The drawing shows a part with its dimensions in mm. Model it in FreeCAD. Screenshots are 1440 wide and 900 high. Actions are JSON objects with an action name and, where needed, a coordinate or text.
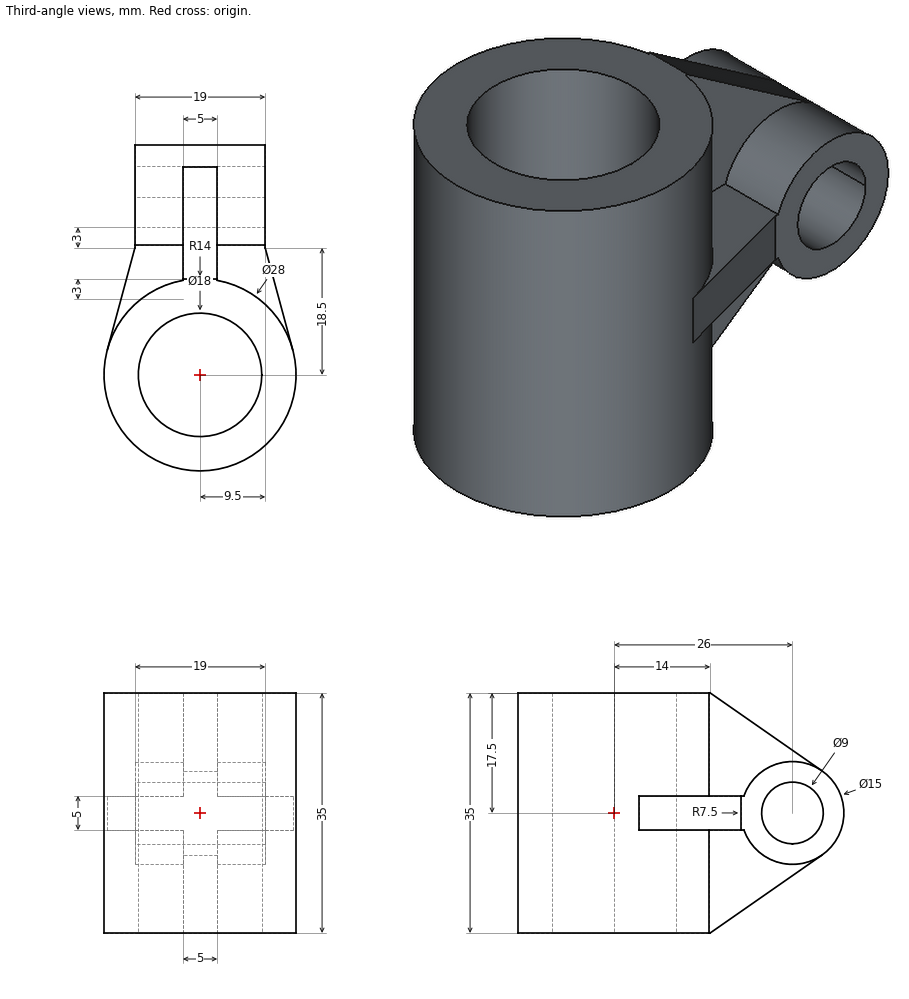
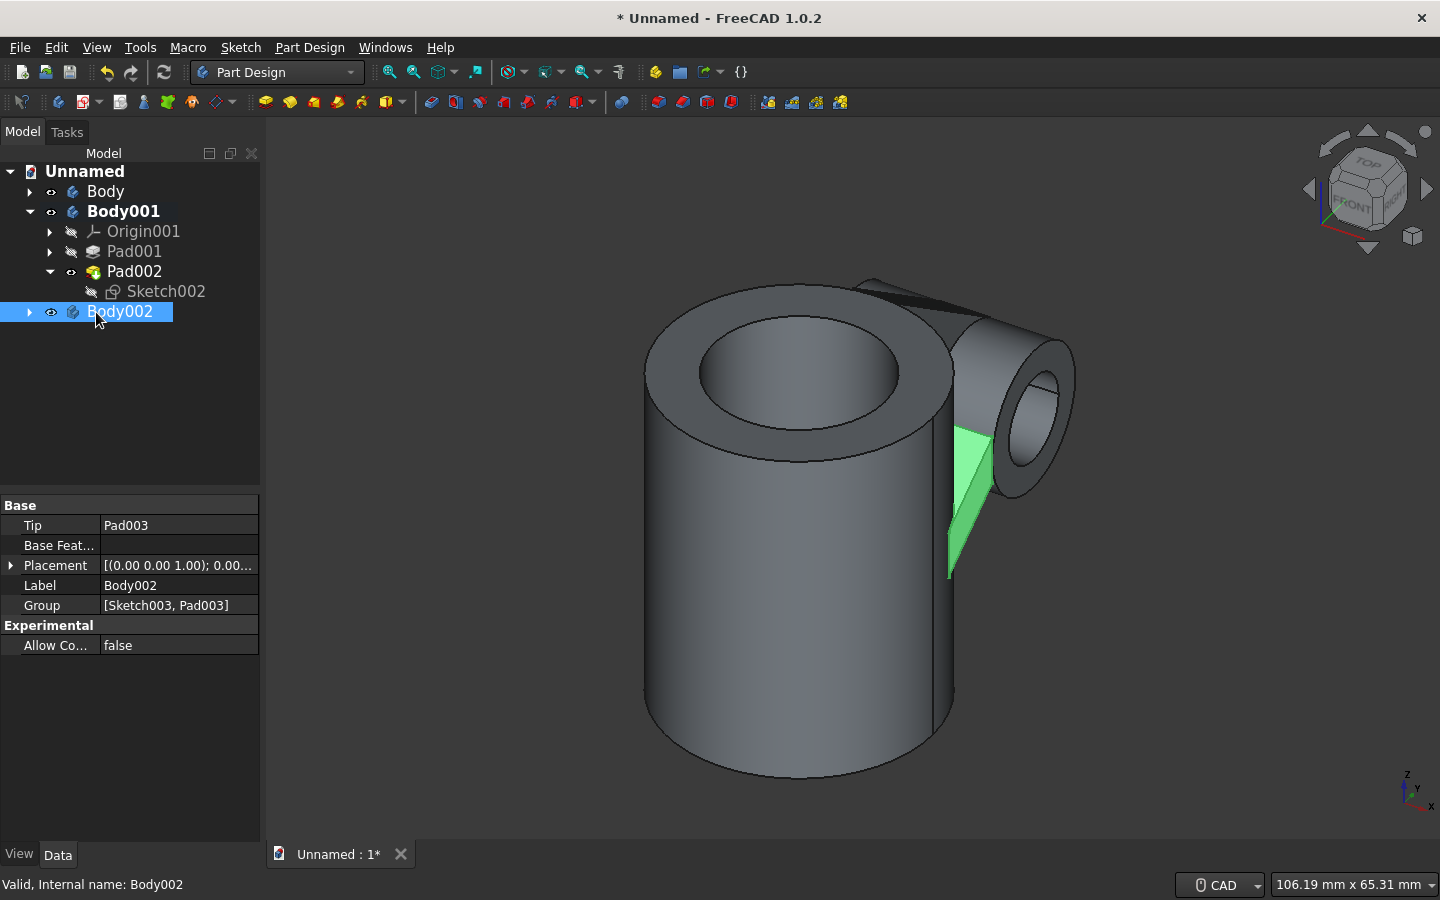
{"action": "left_click", "coordinate": [622, 102]}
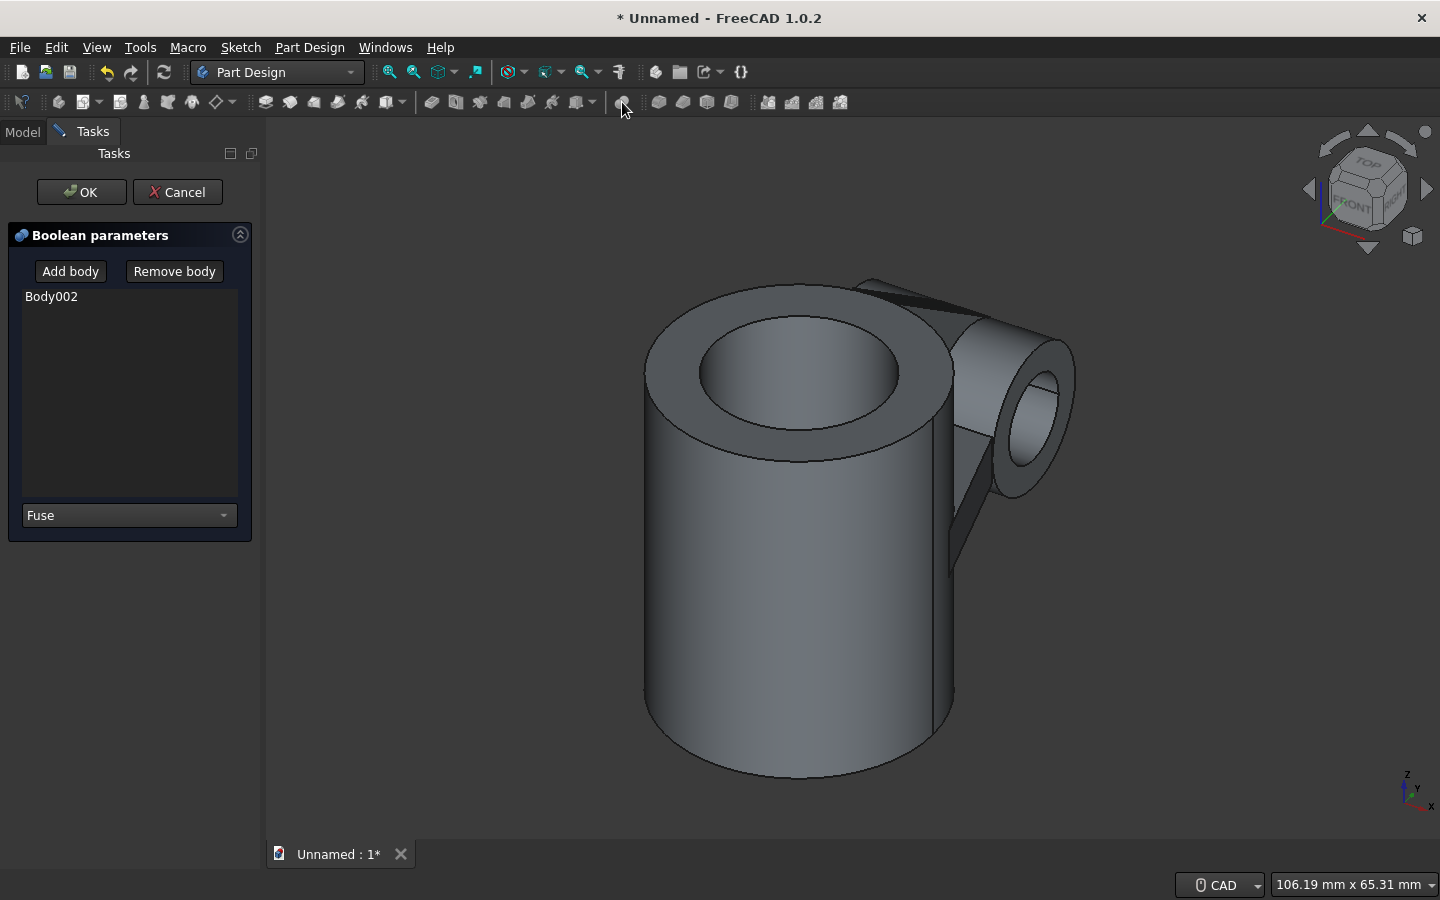
{"action": "left_click", "coordinate": [82, 192]}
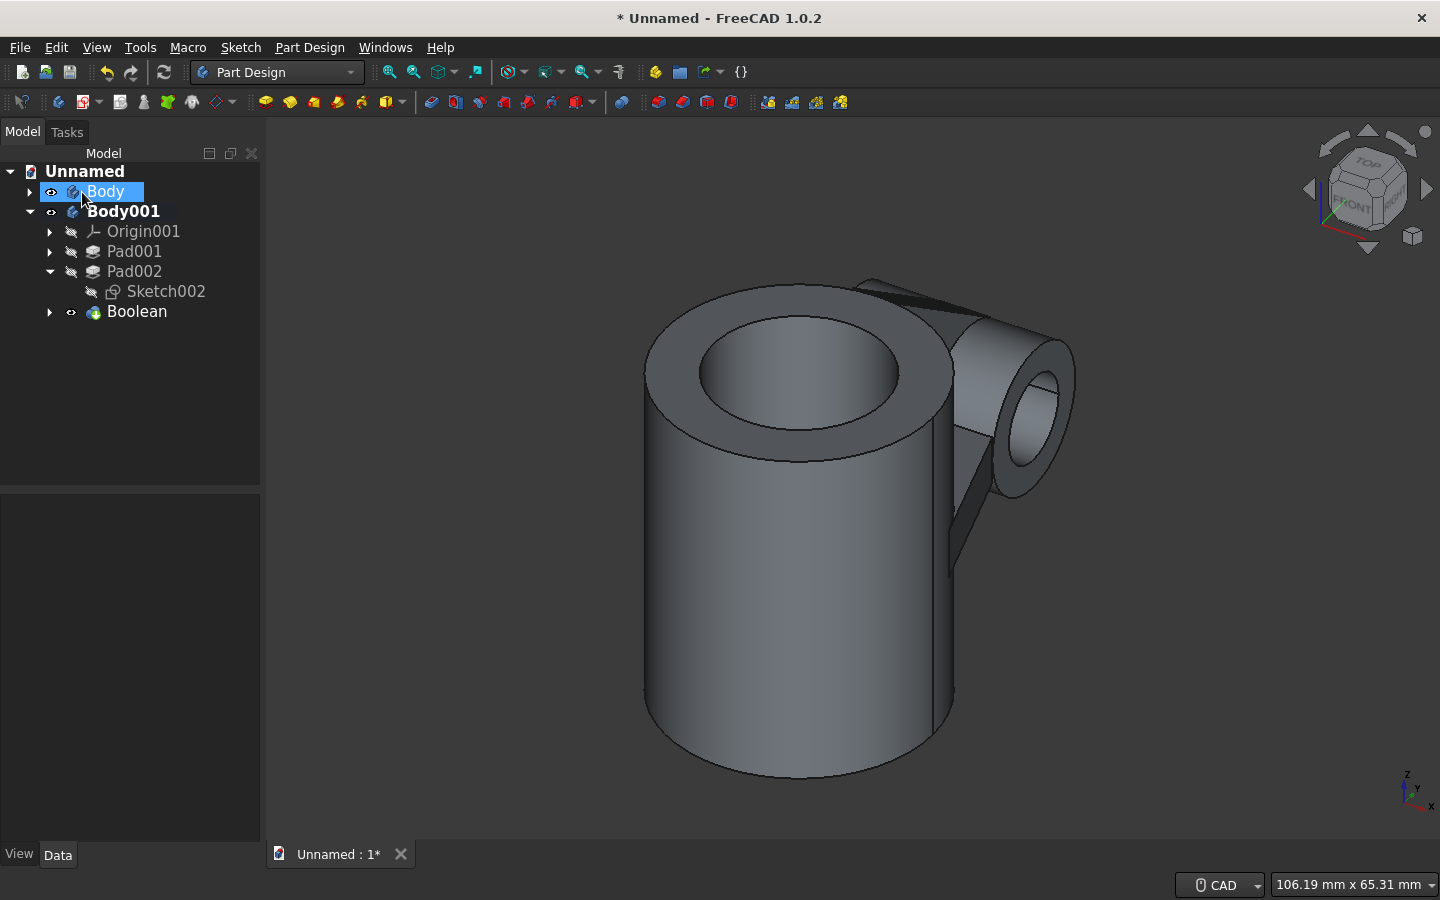
{"action": "left_click", "coordinate": [50, 232]}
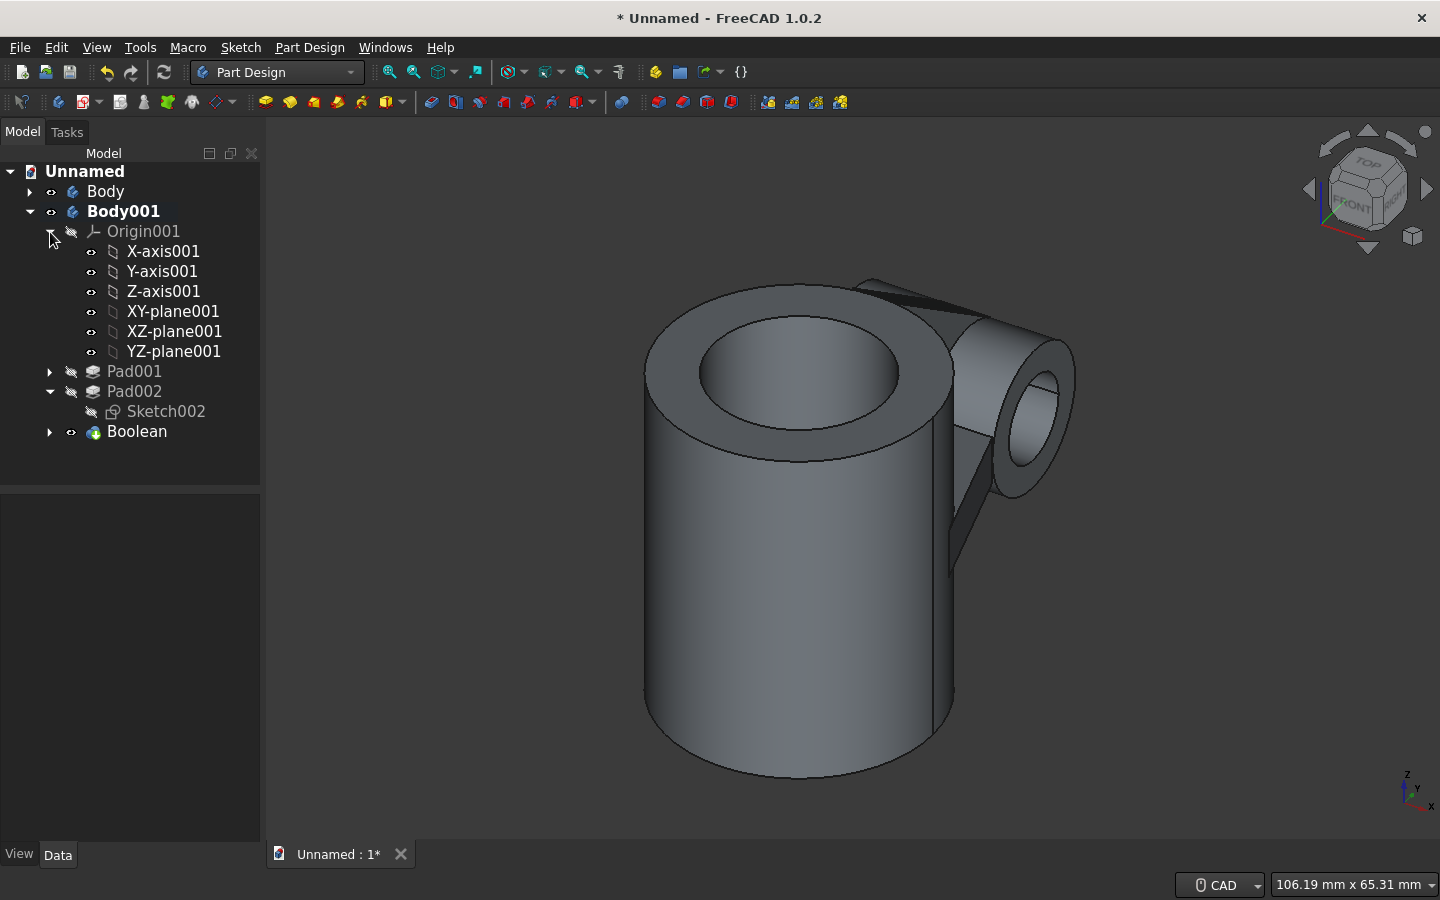
{"action": "left_click", "coordinate": [136, 332]}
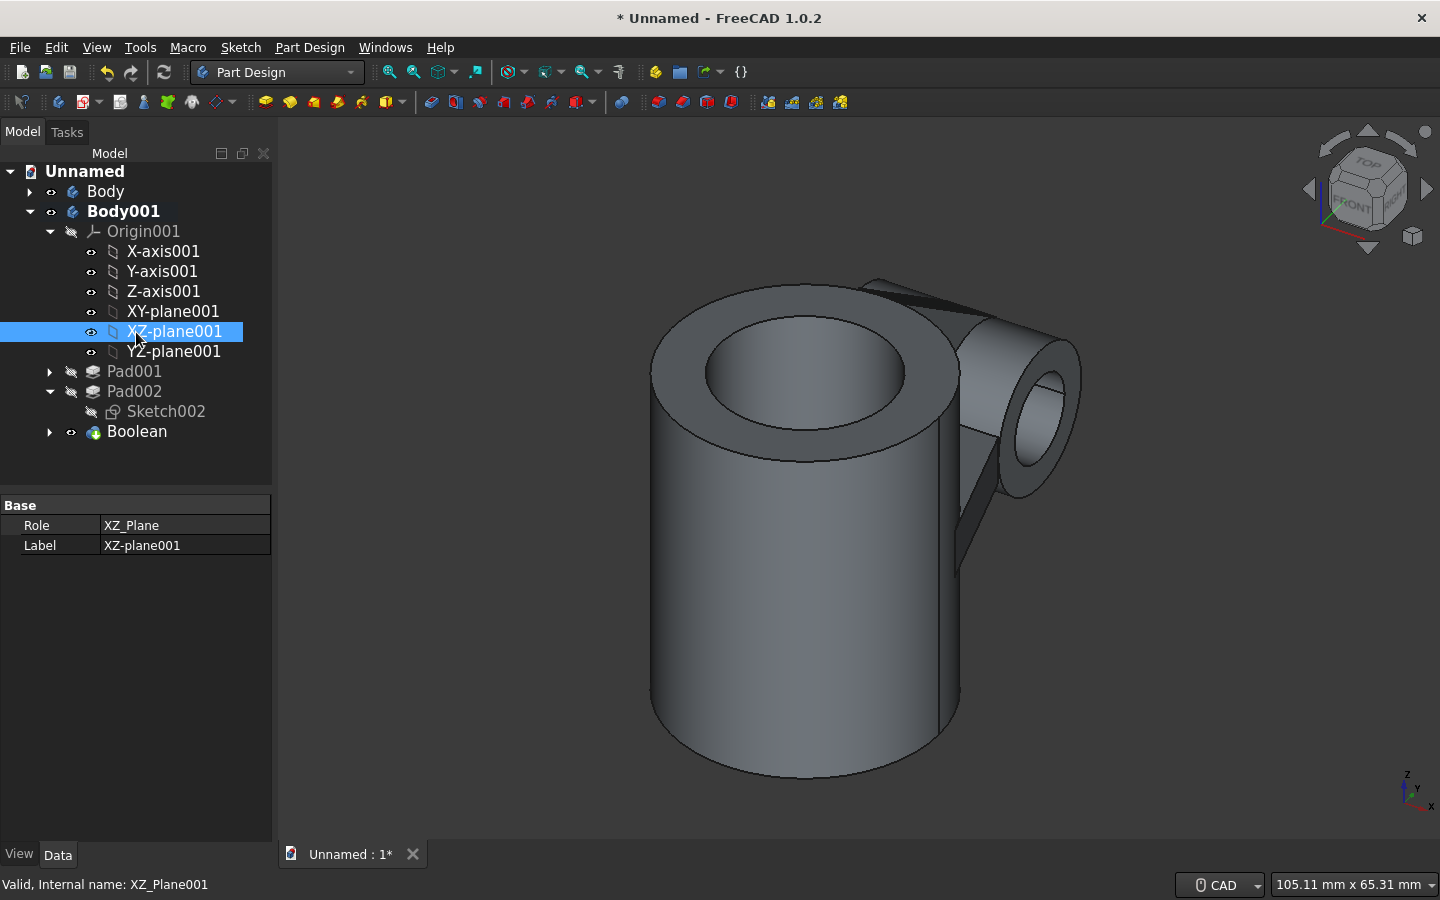
{"action": "left_click", "coordinate": [216, 102]}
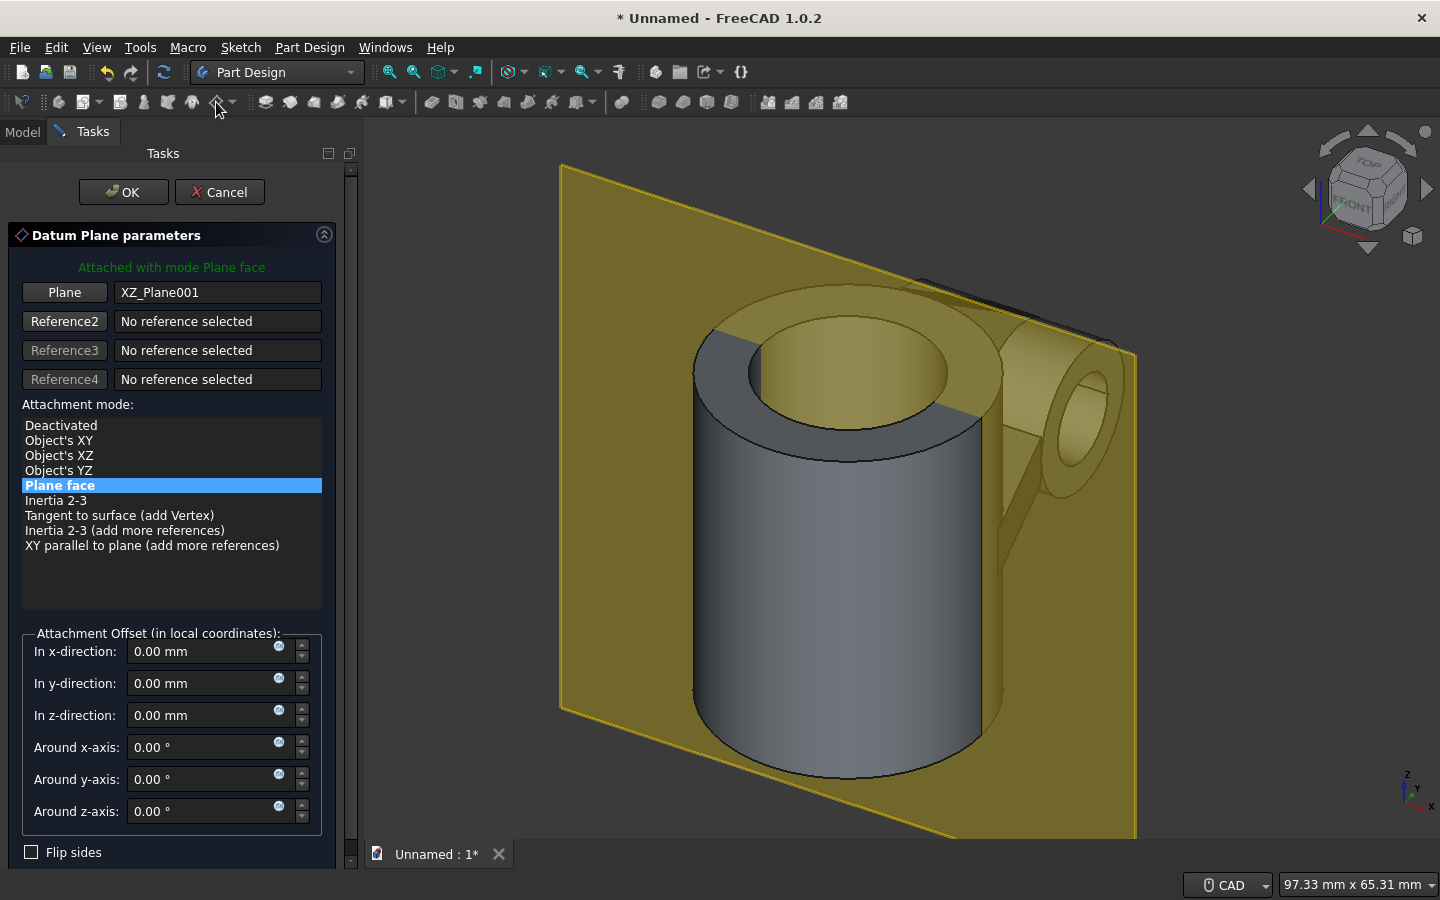
{"action": "triple_click", "coordinate": [210, 715]}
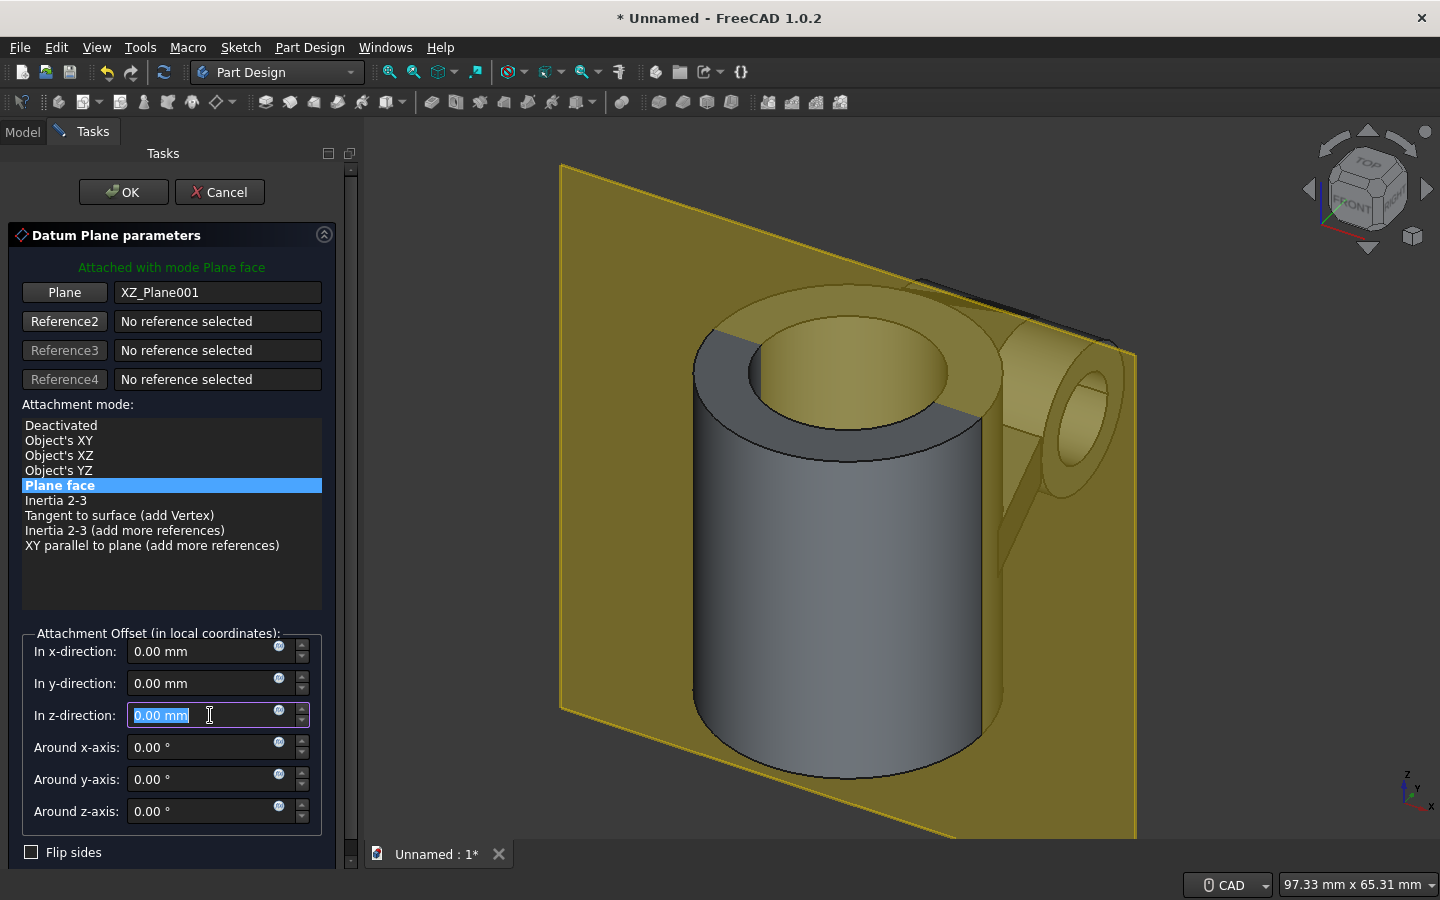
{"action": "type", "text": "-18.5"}
{"action": "key", "text": "Tab"}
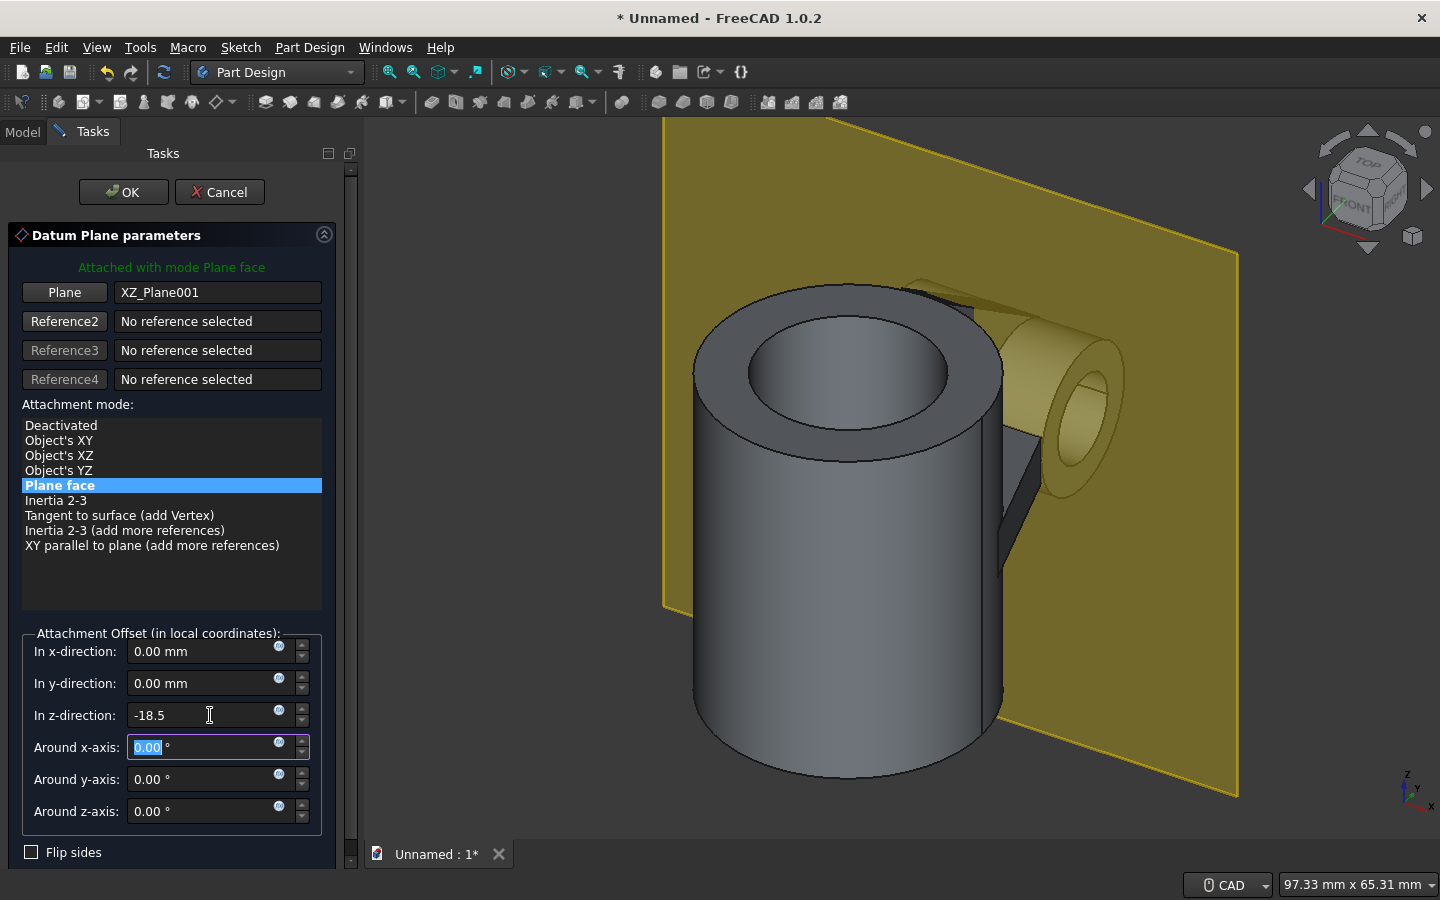
{"action": "left_click", "coordinate": [124, 192]}